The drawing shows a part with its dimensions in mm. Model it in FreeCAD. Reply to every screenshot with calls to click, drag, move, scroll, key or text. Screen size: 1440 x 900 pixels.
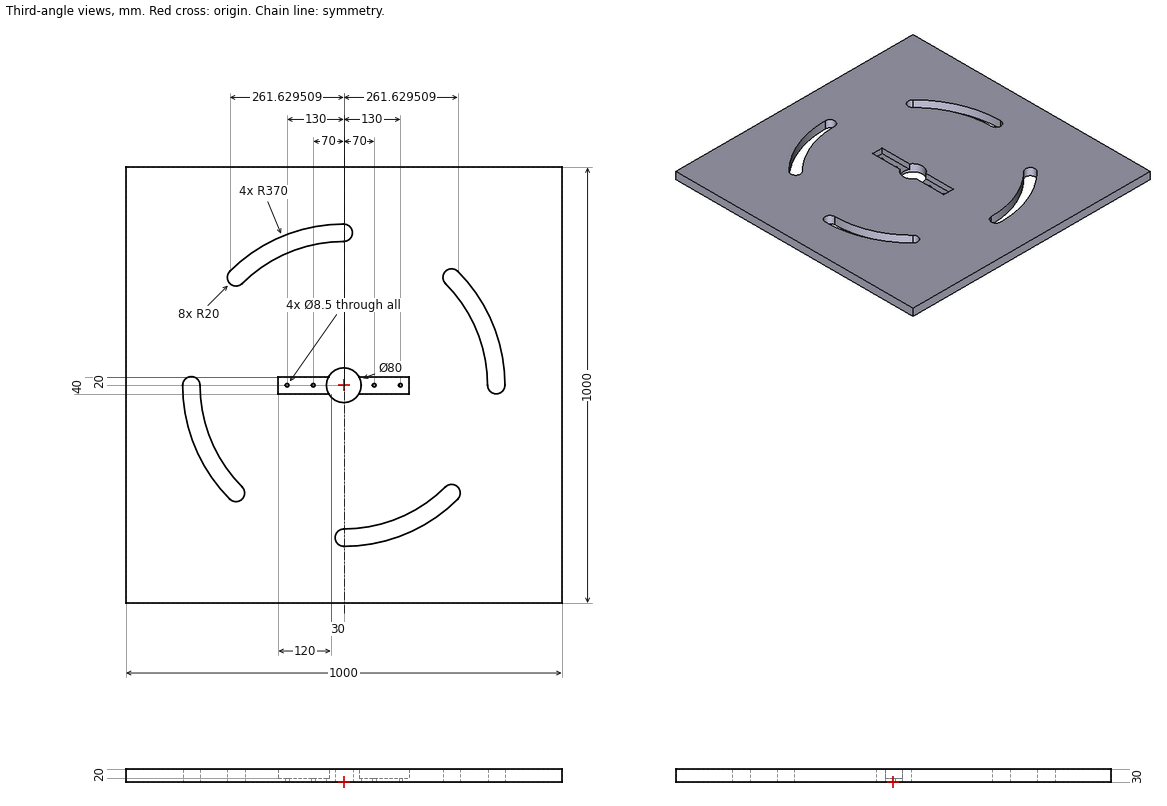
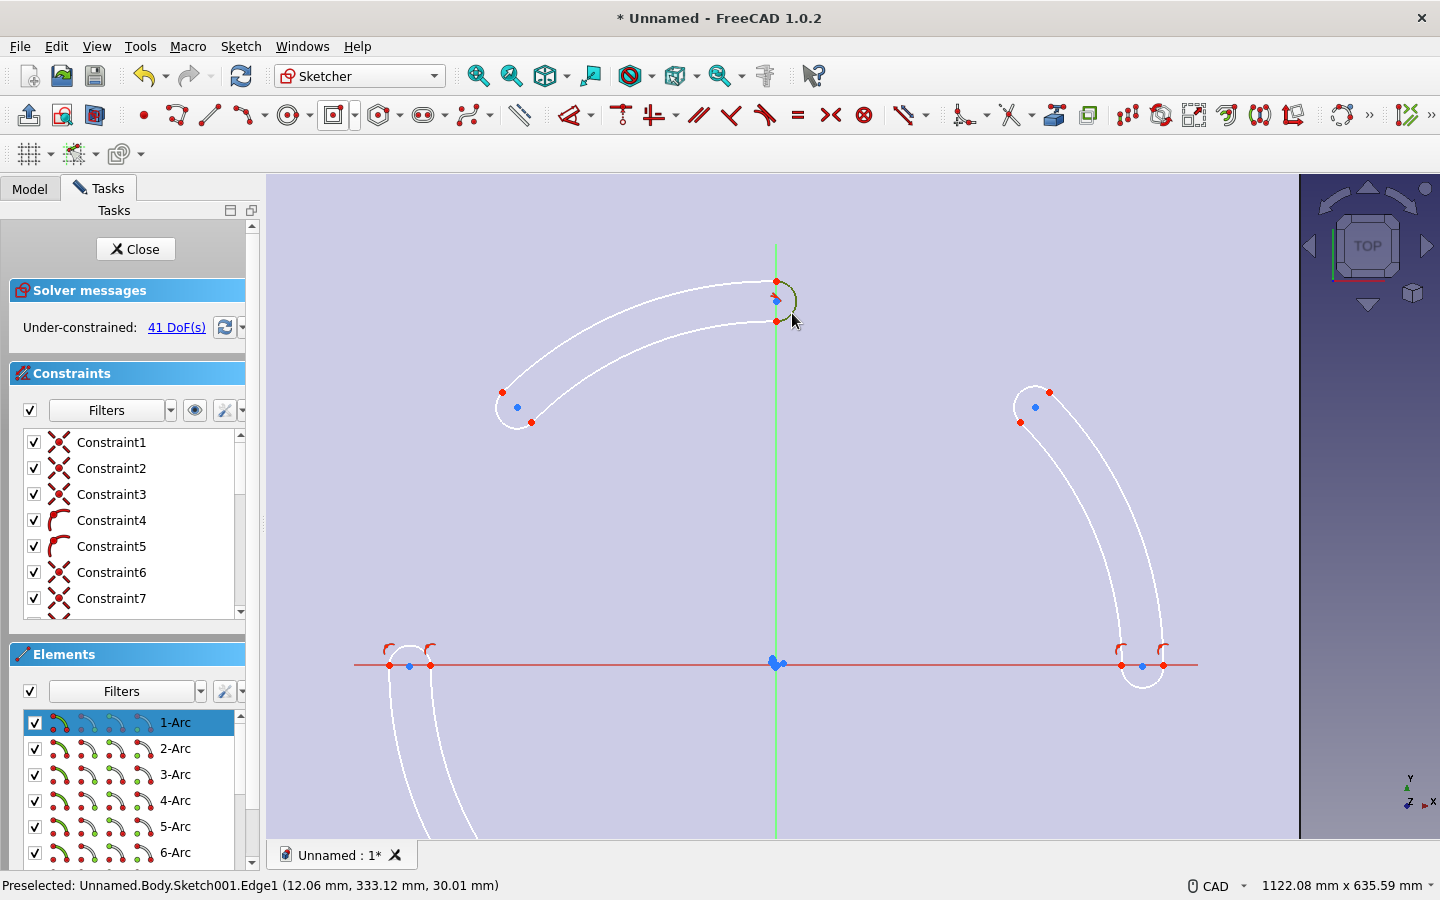
click(696, 331)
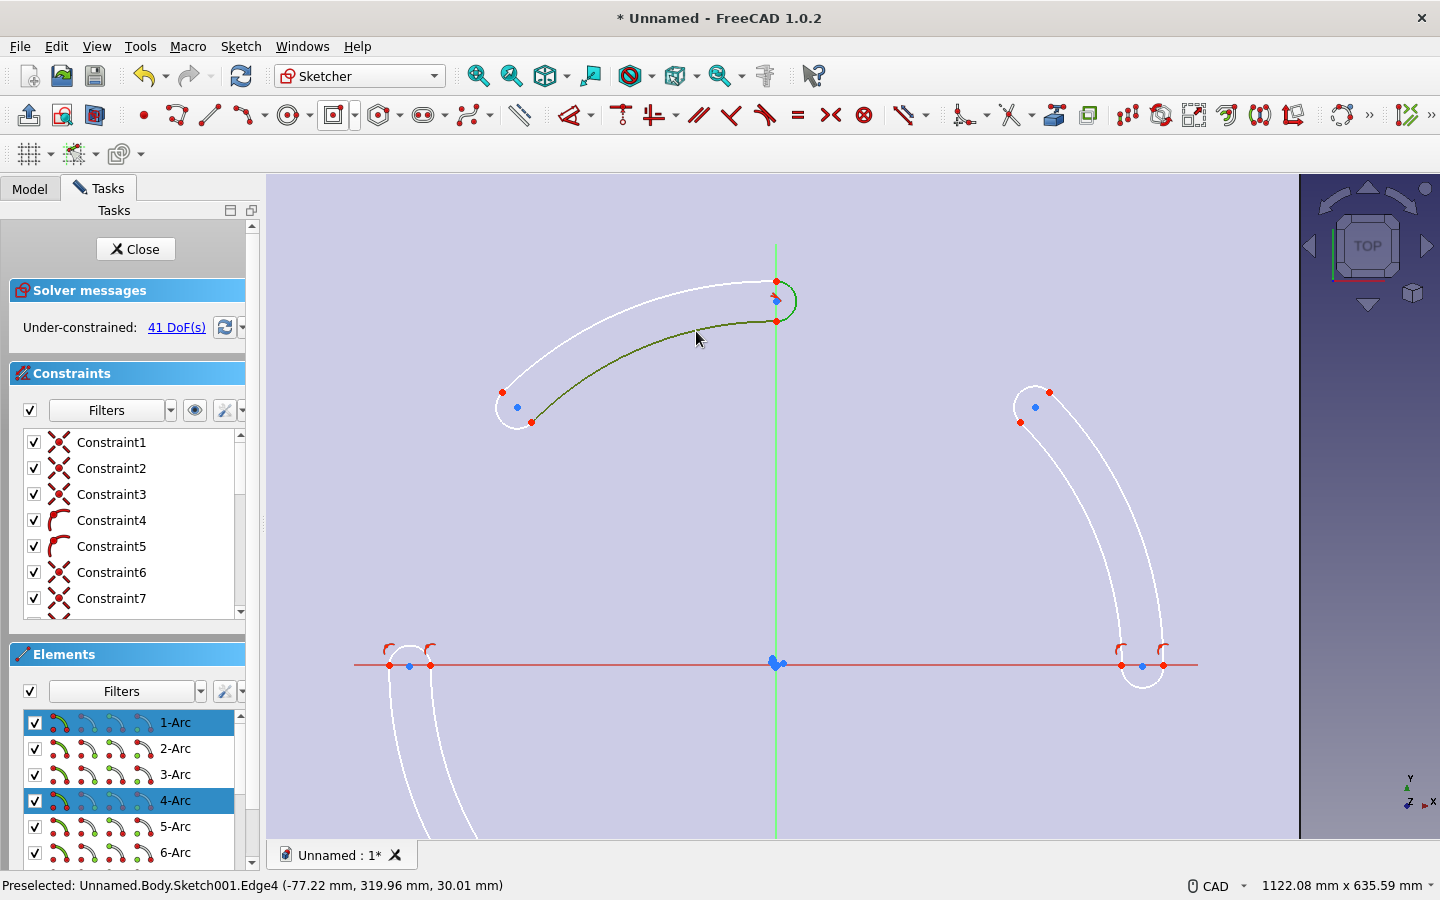
click(765, 116)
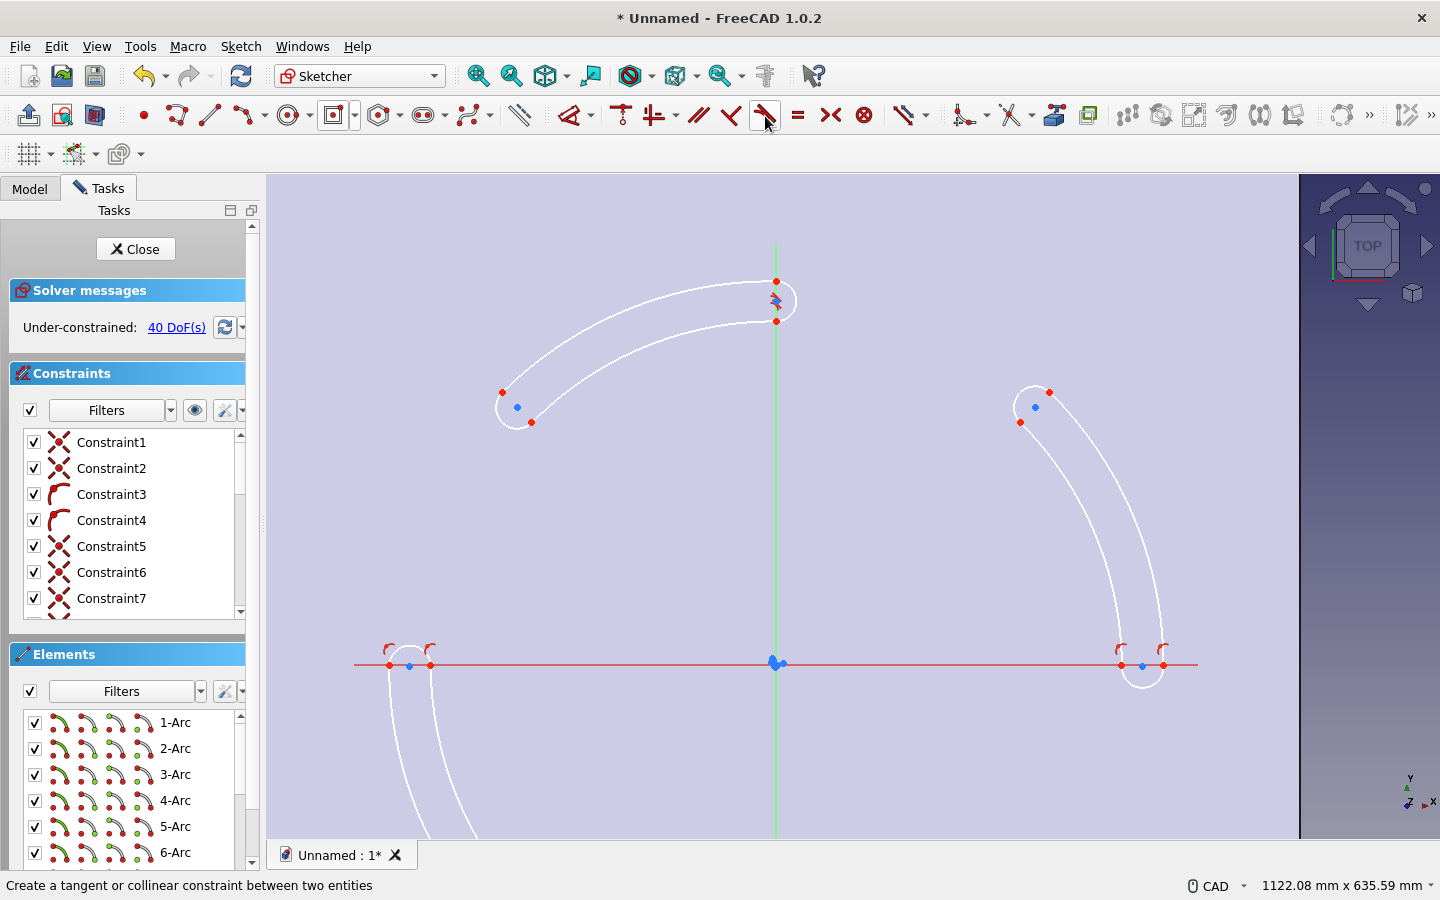
click(686, 291)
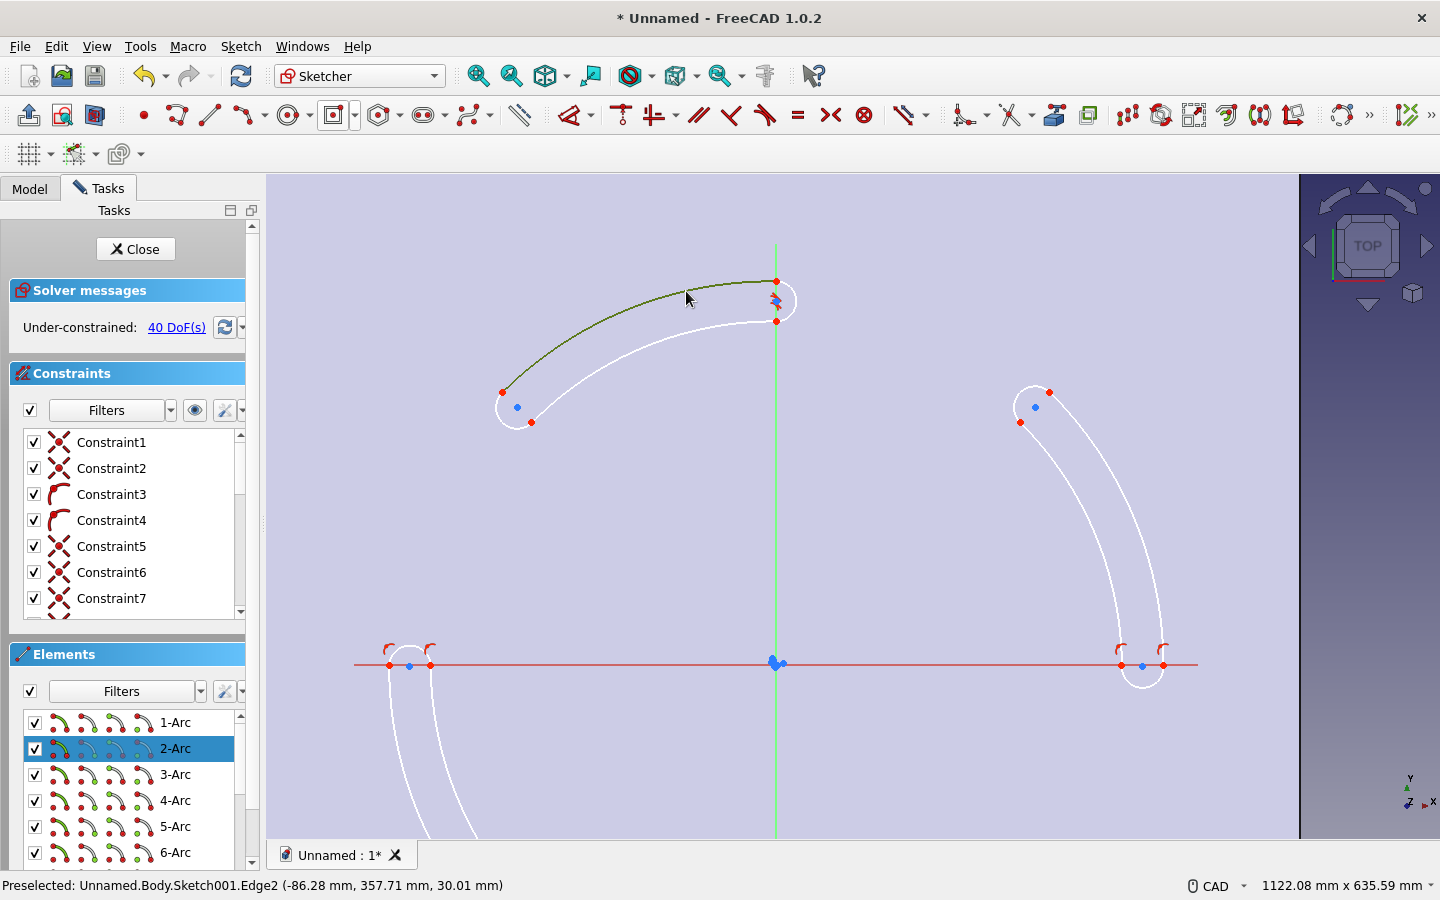
click(496, 410)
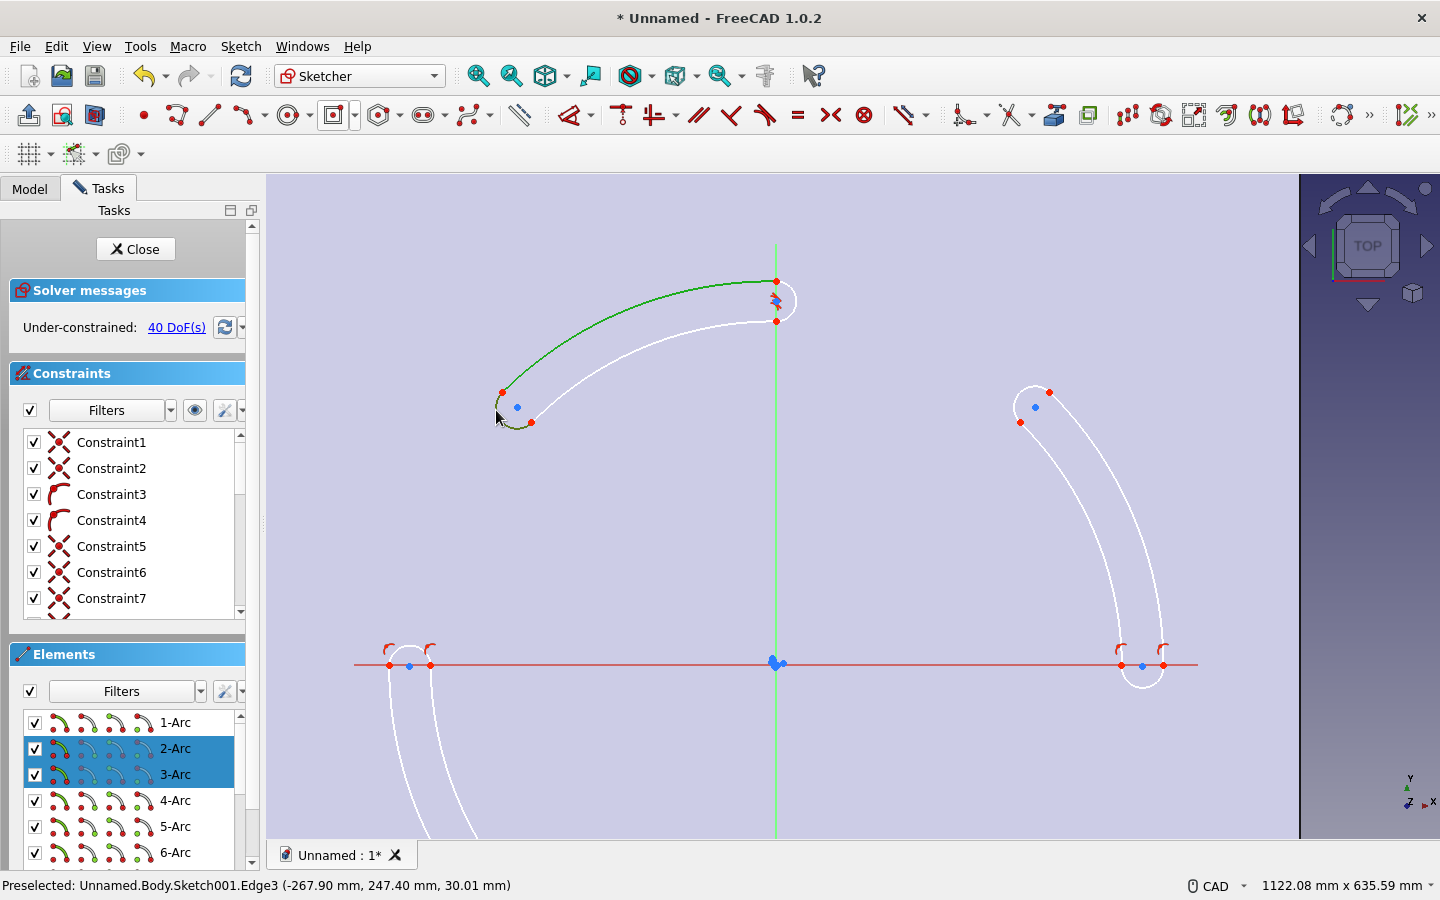
click(765, 116)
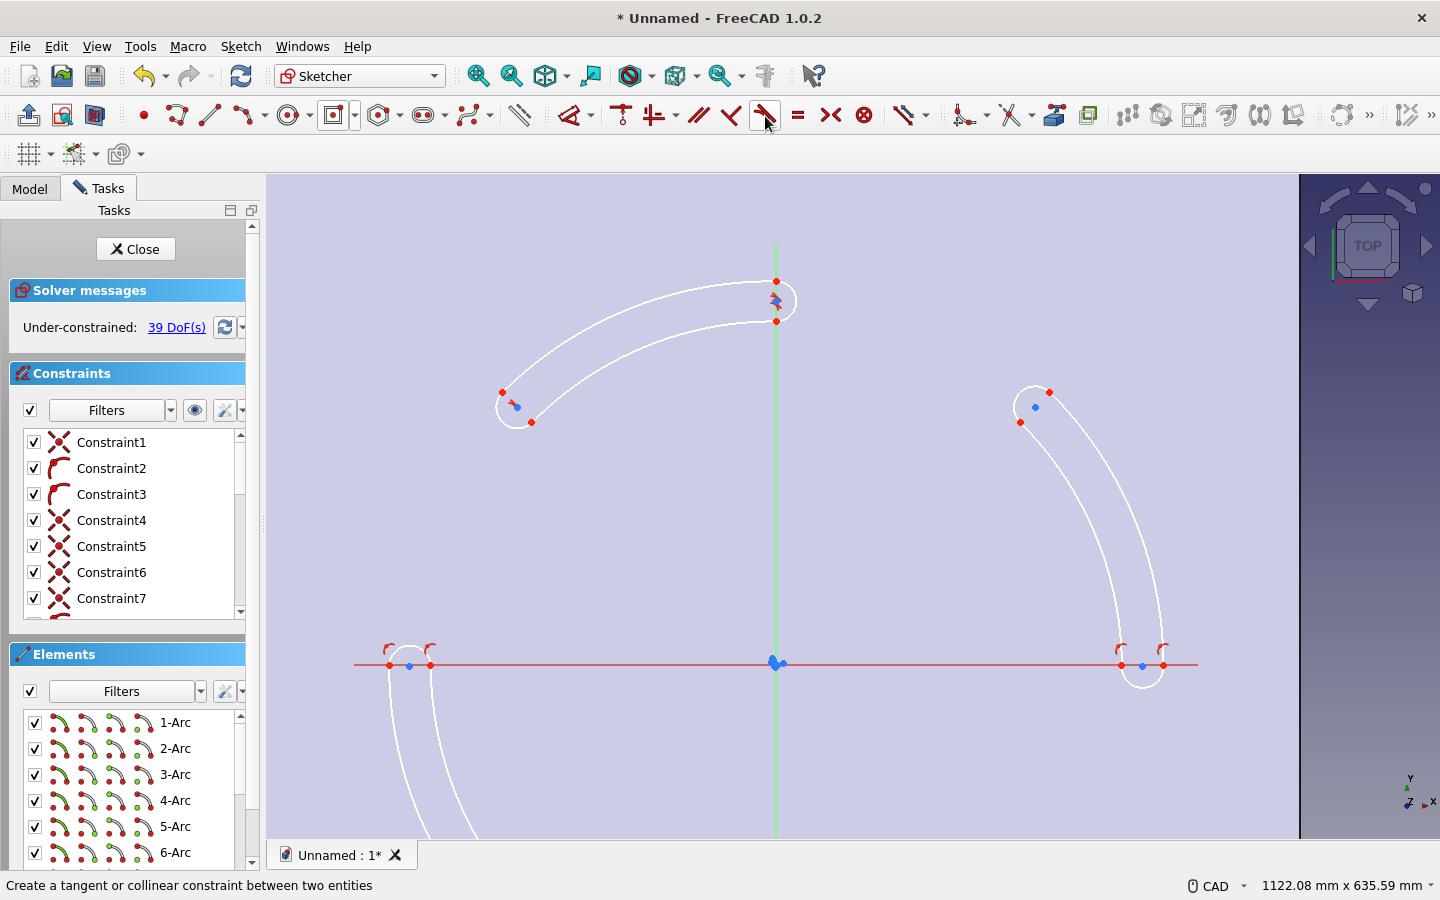
click(497, 410)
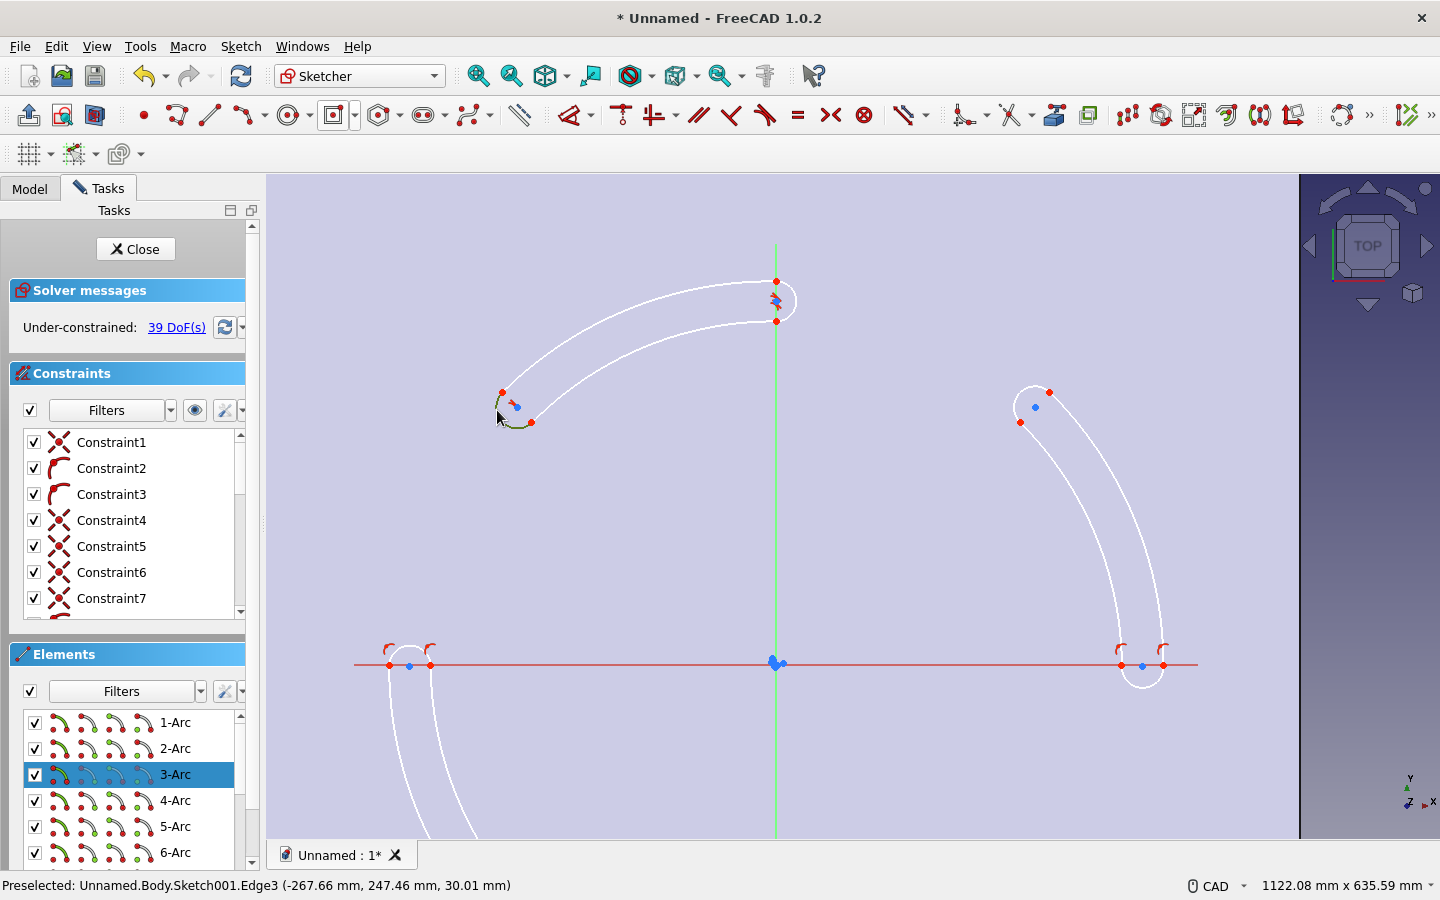
click(695, 331)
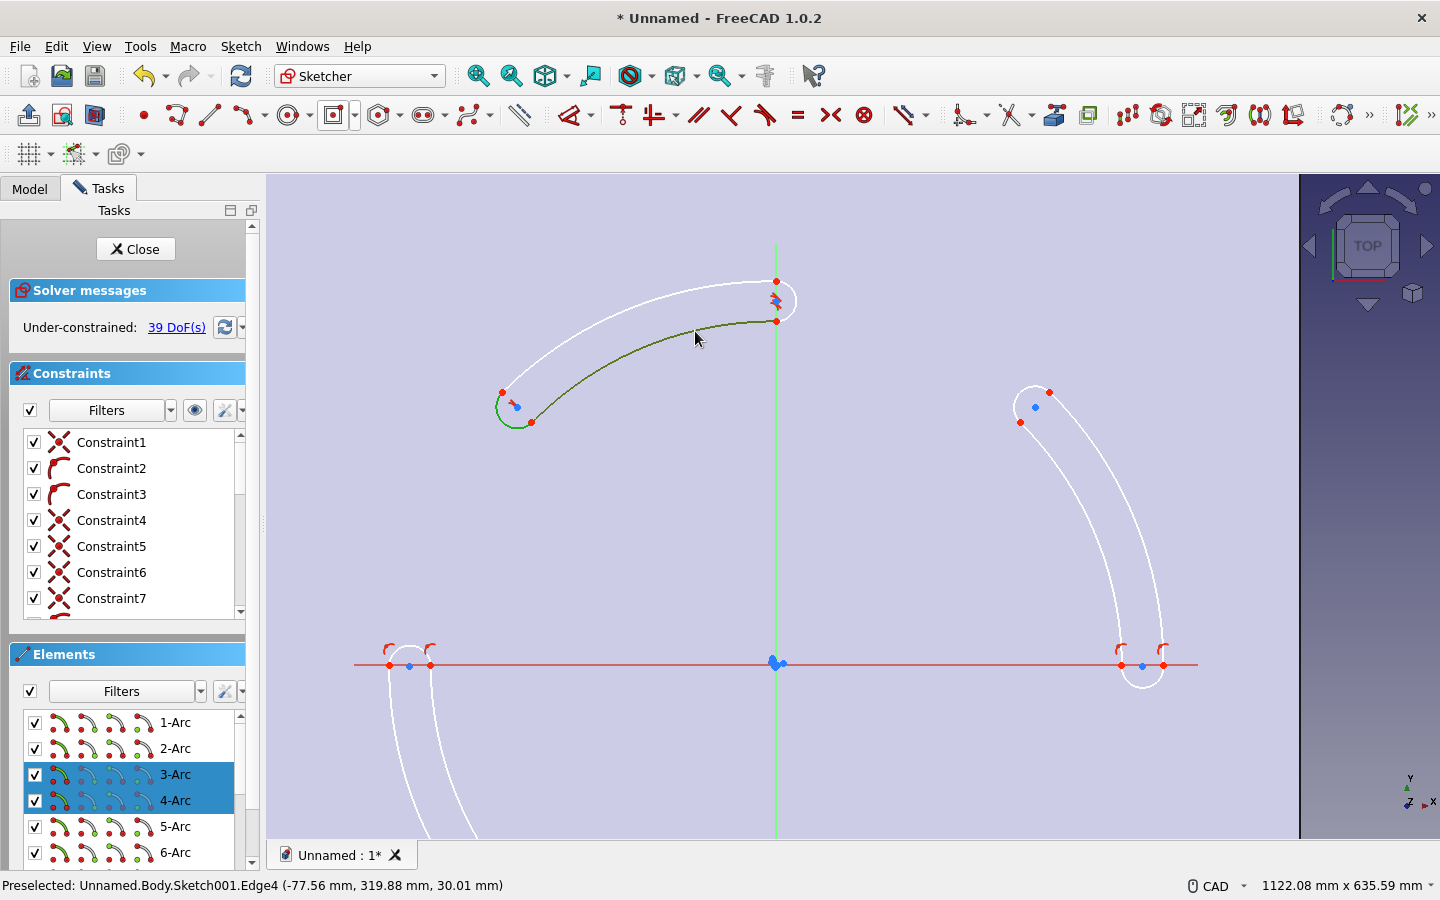
key(t)